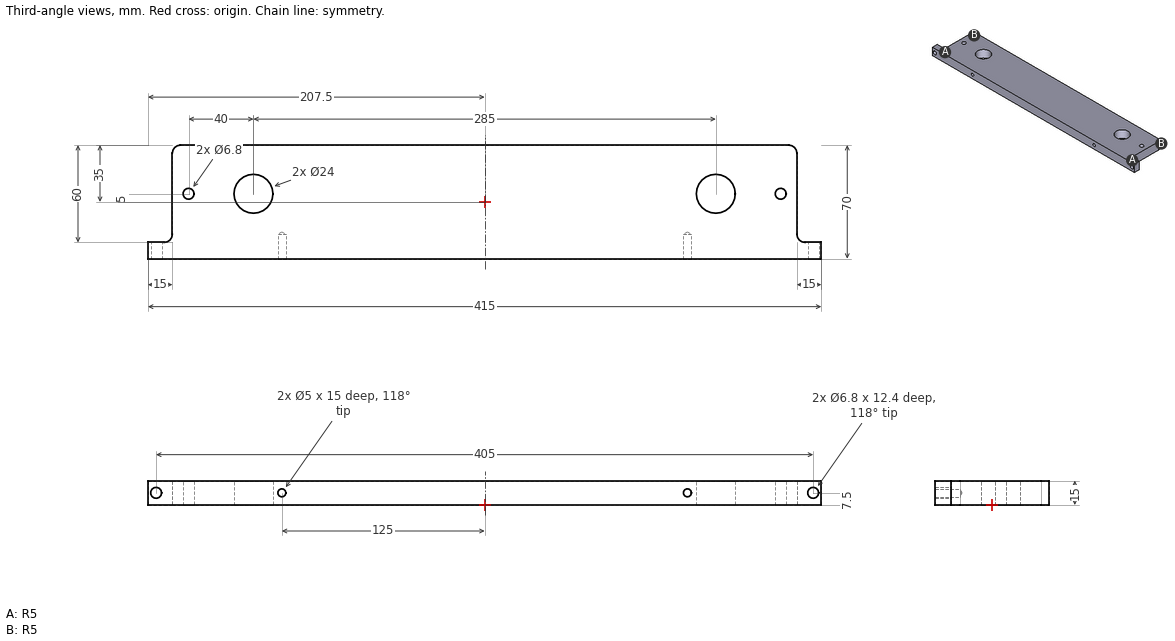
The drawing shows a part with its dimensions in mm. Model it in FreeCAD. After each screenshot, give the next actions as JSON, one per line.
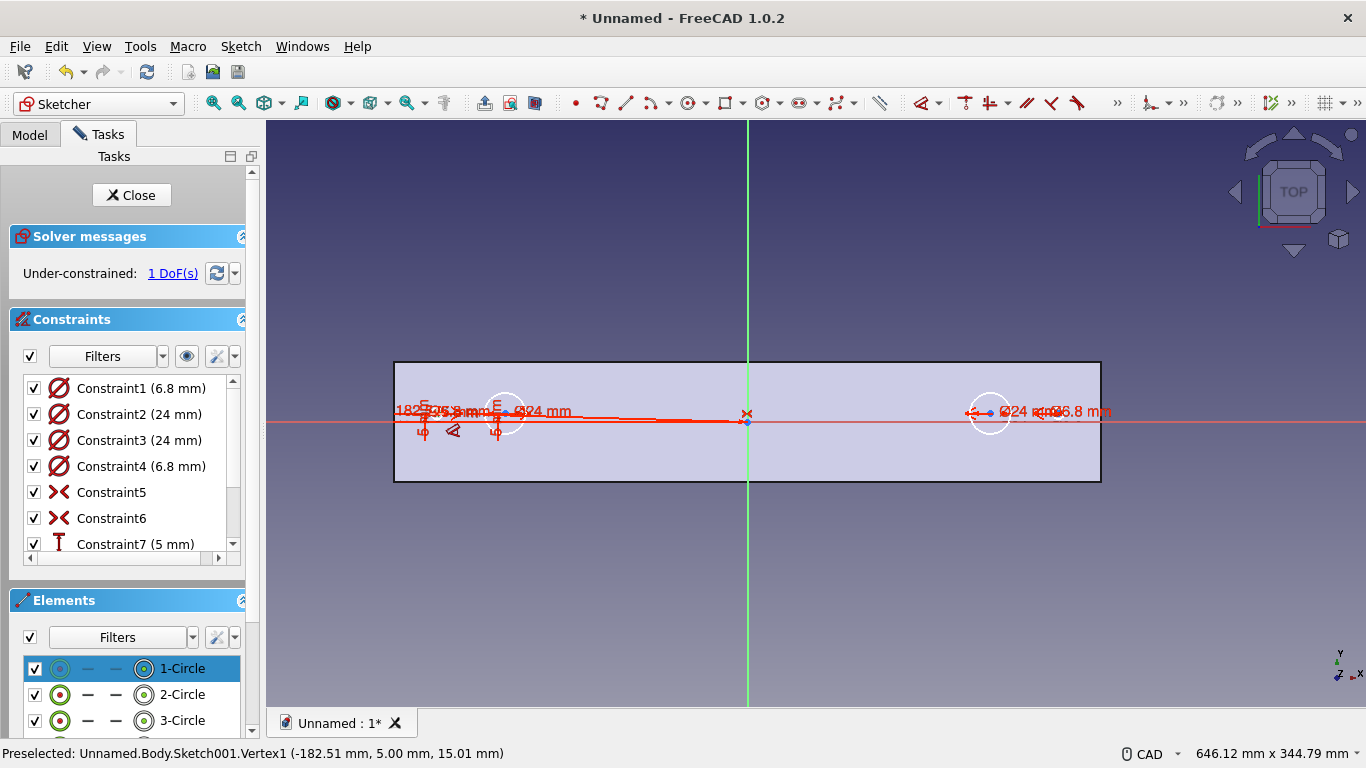
{"action": "left_click", "coordinate": [505, 414]}
{"action": "left_click", "coordinate": [471, 448]}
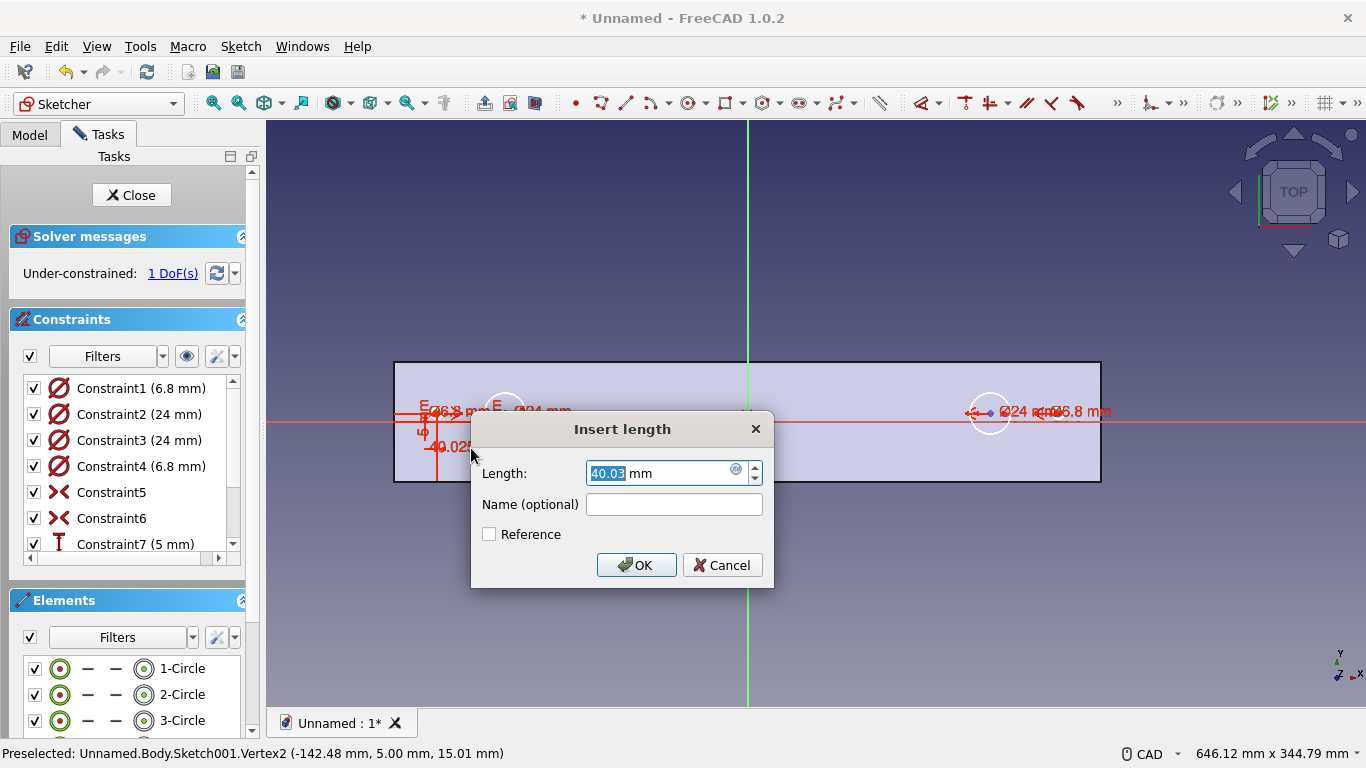
{"action": "type", "text": "40"}
{"action": "key", "text": "Return"}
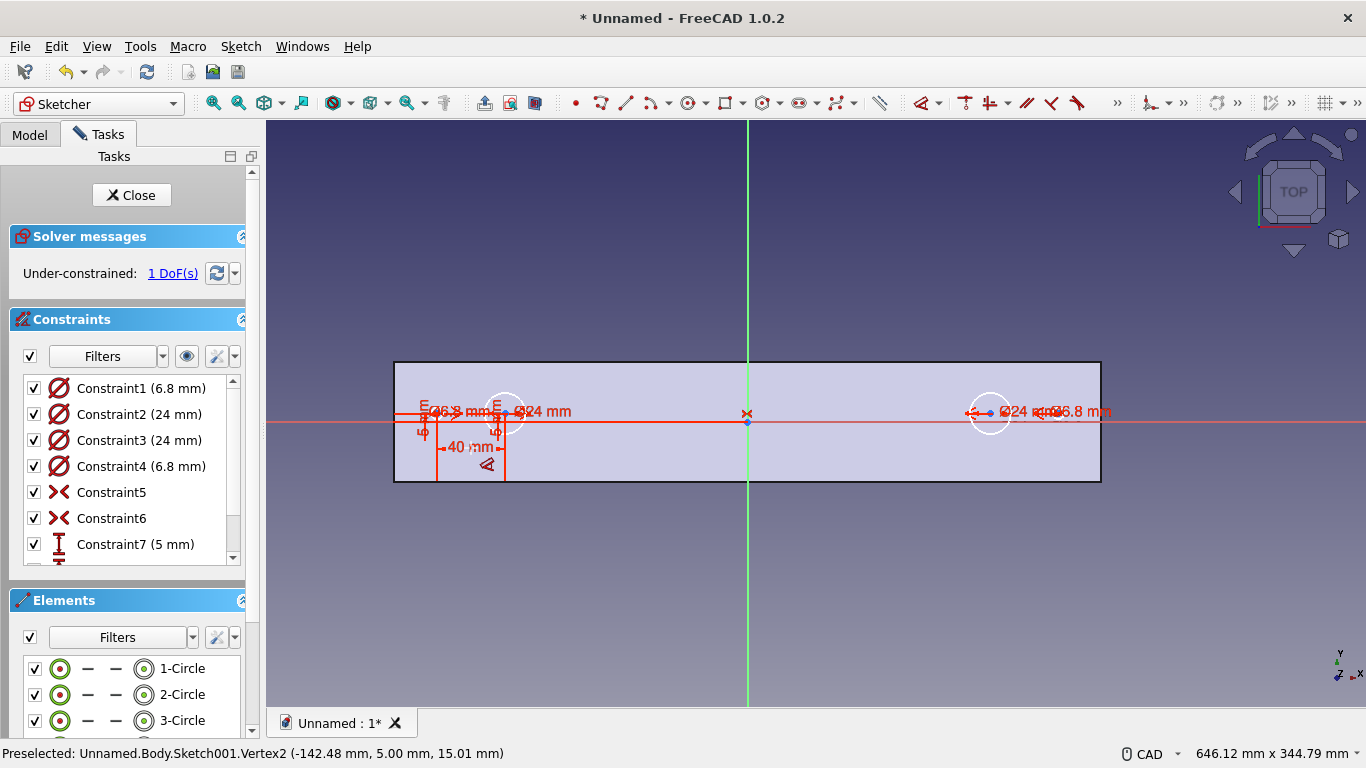
{"action": "left_click", "coordinate": [505, 414]}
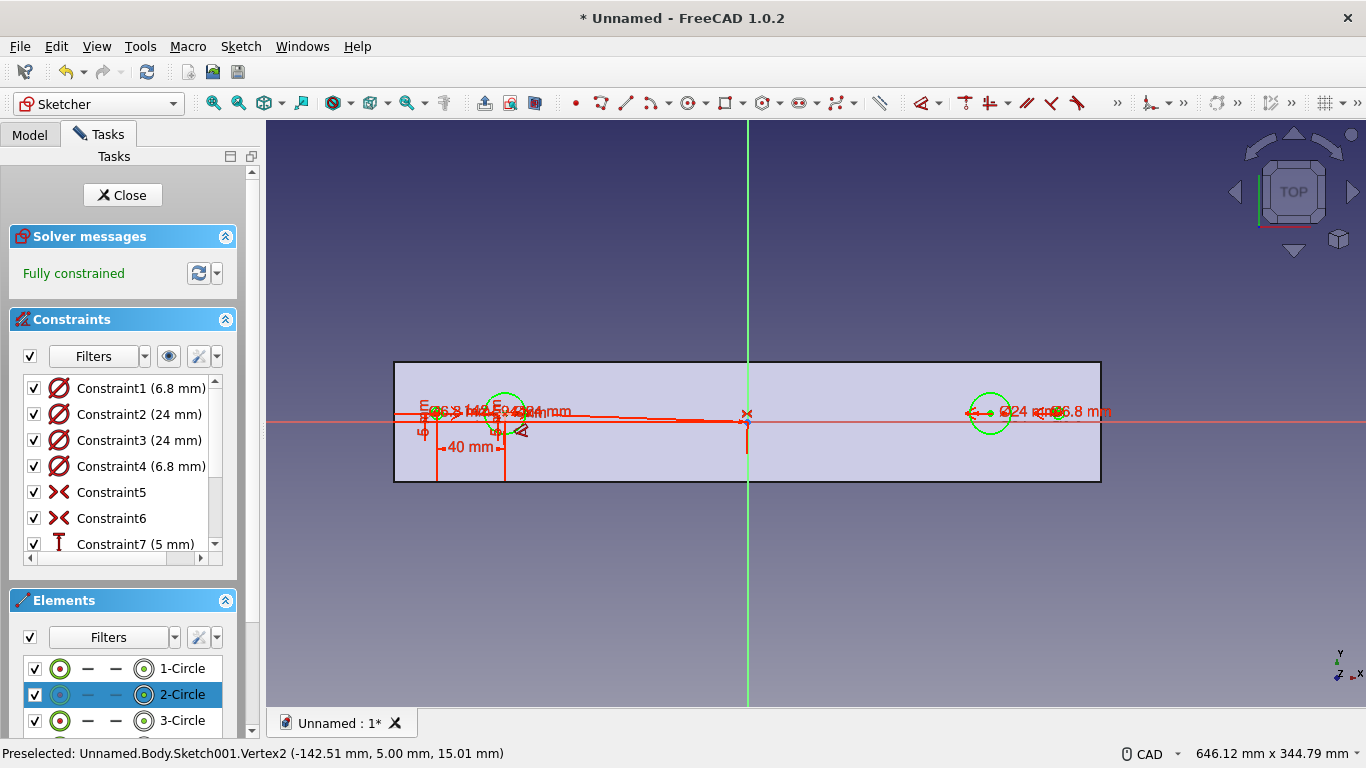
{"action": "left_click", "coordinate": [990, 414]}
{"action": "left_click", "coordinate": [636, 448]}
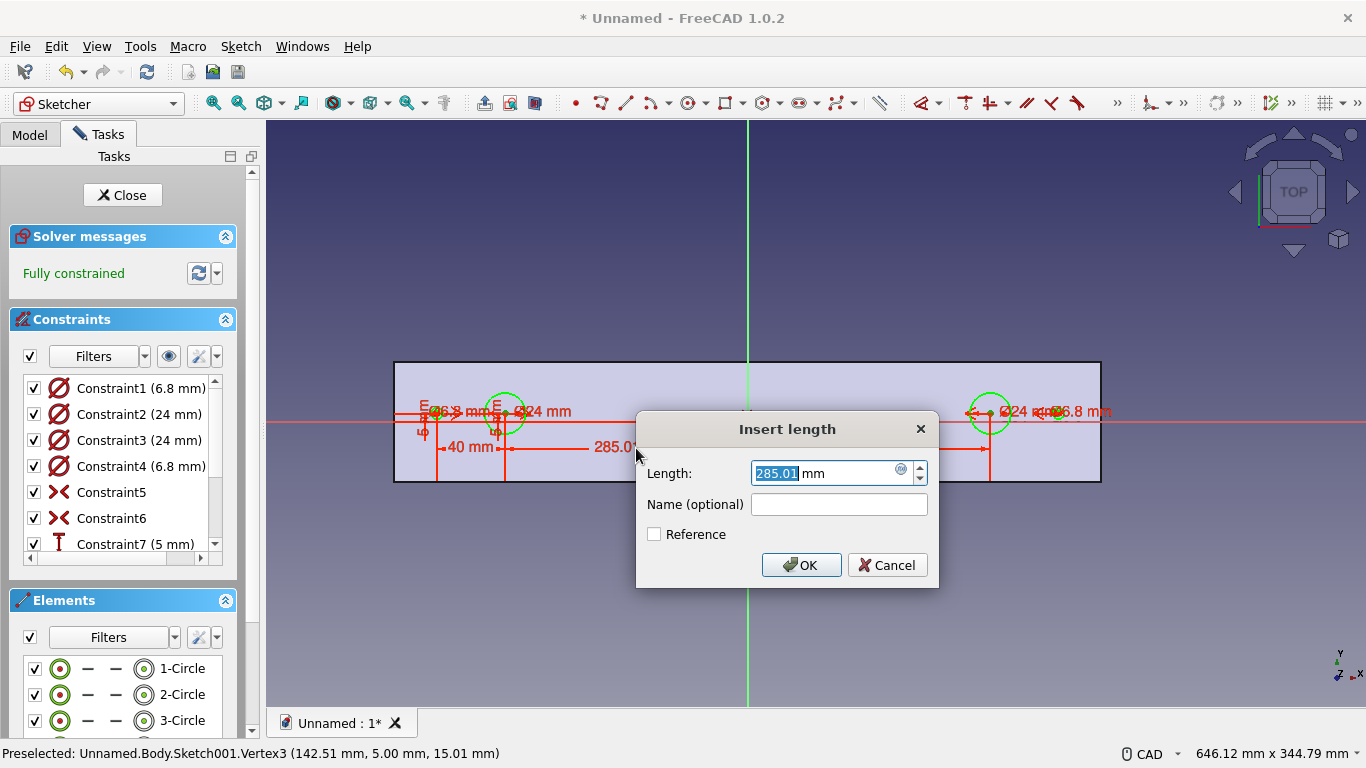
{"action": "type", "text": "285"}
{"action": "key", "text": "Return"}
{"action": "key", "text": "Escape"}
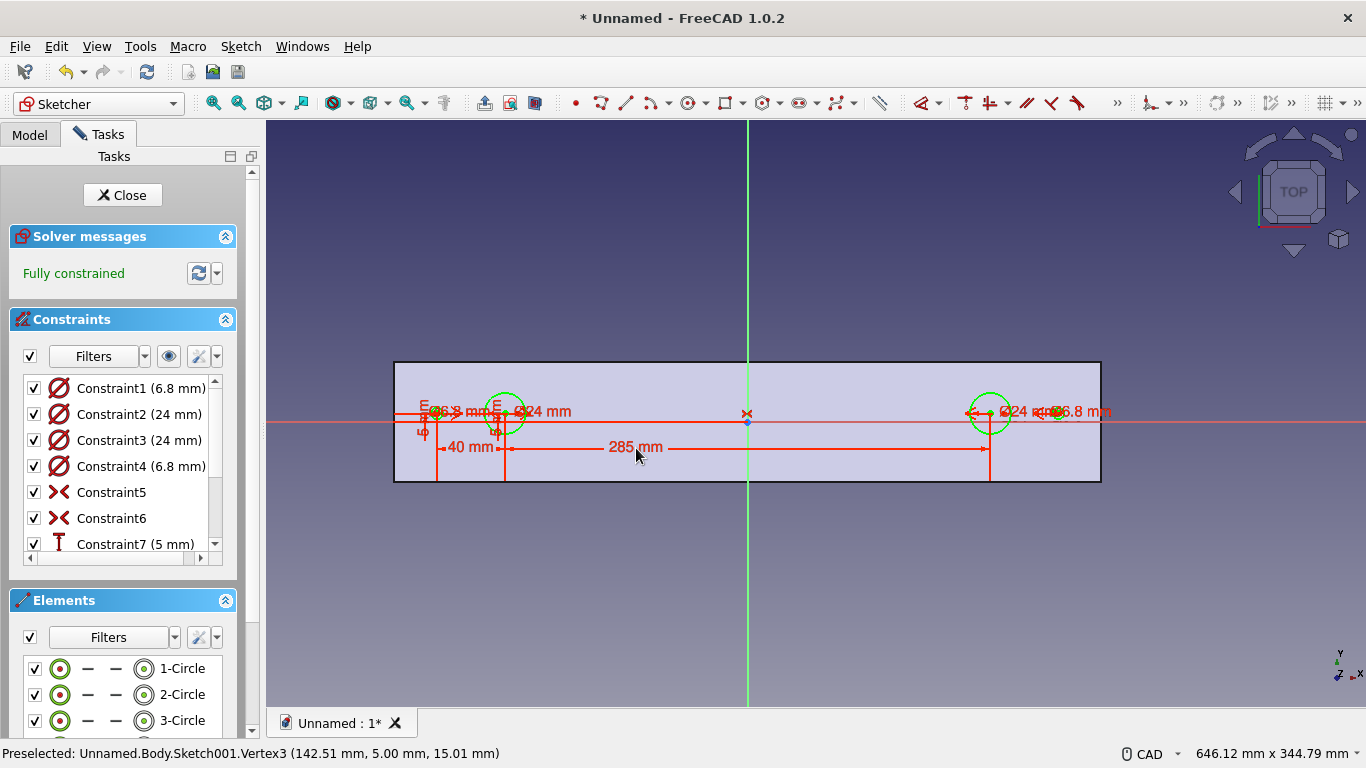
{"action": "left_click", "coordinate": [123, 195]}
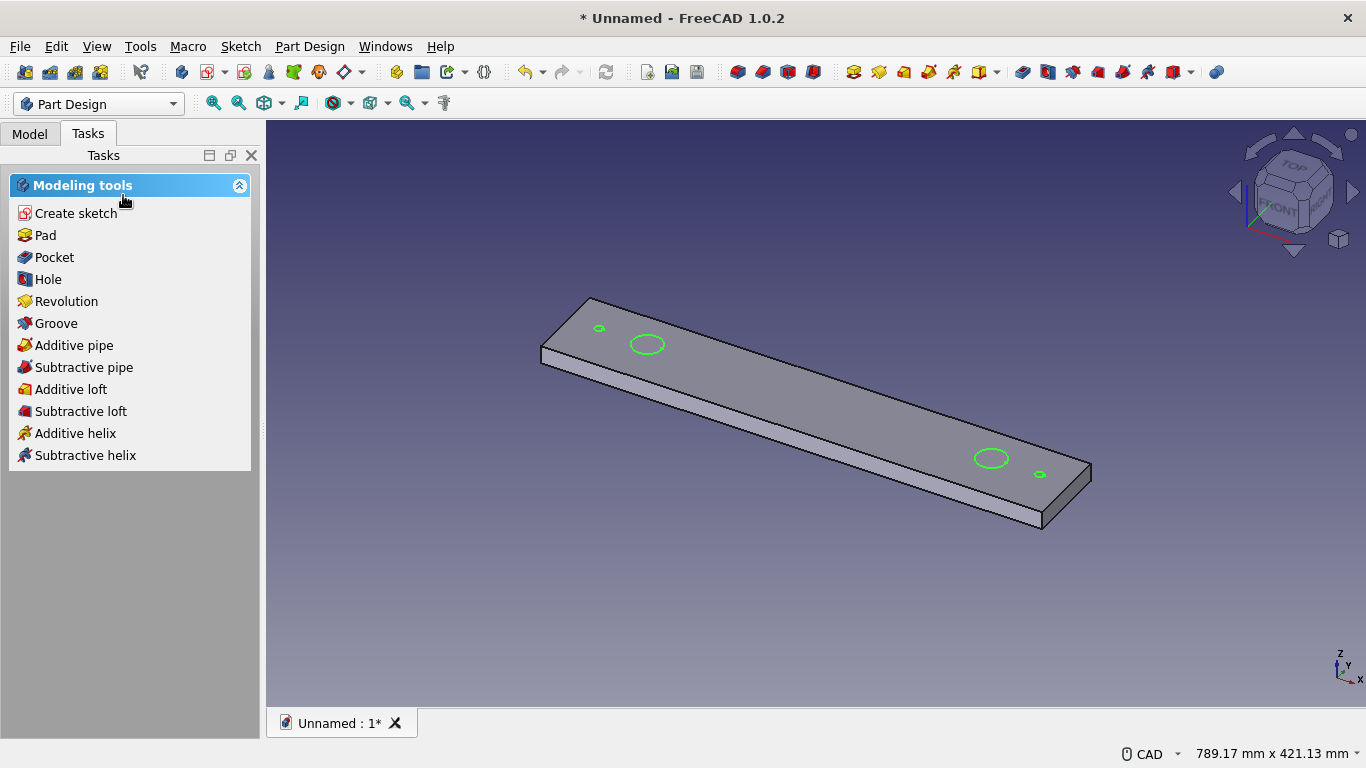
{"action": "left_click", "coordinate": [1023, 72]}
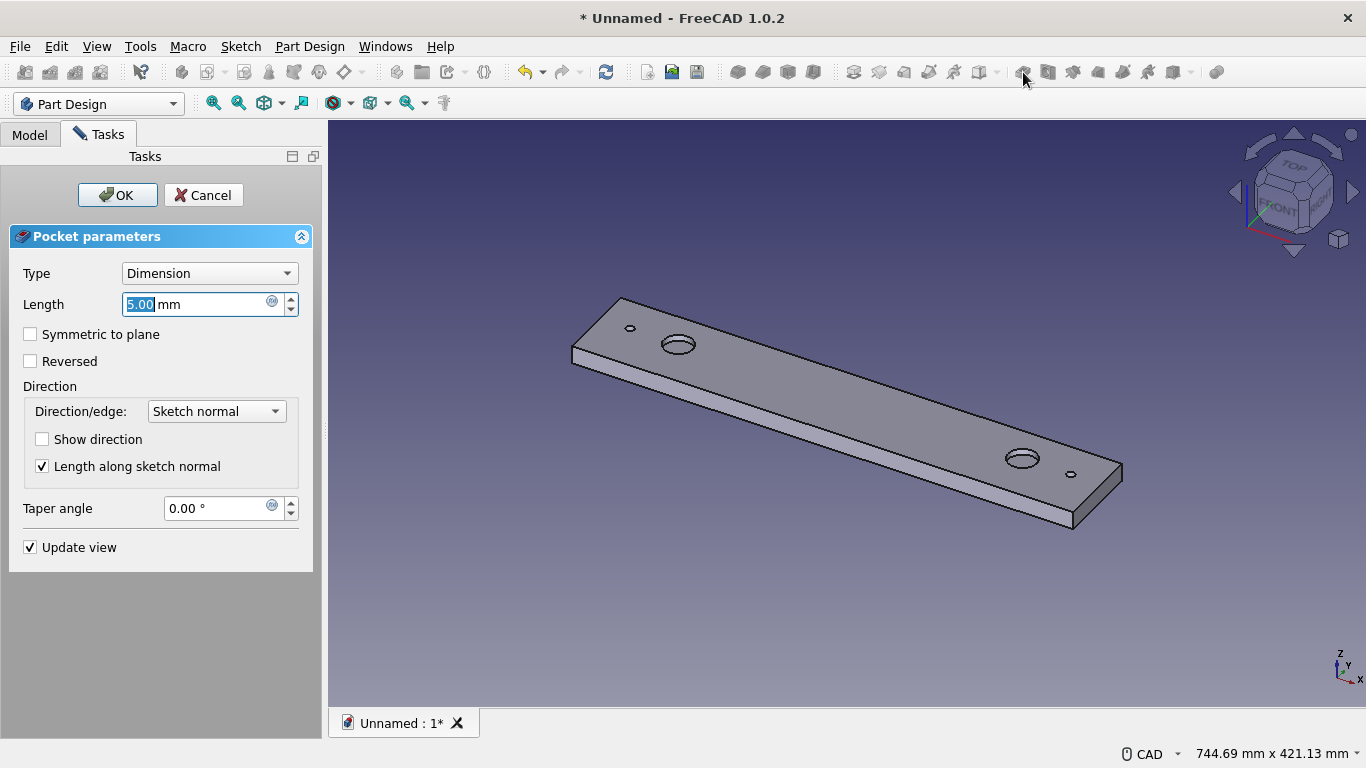
{"action": "left_click", "coordinate": [210, 274]}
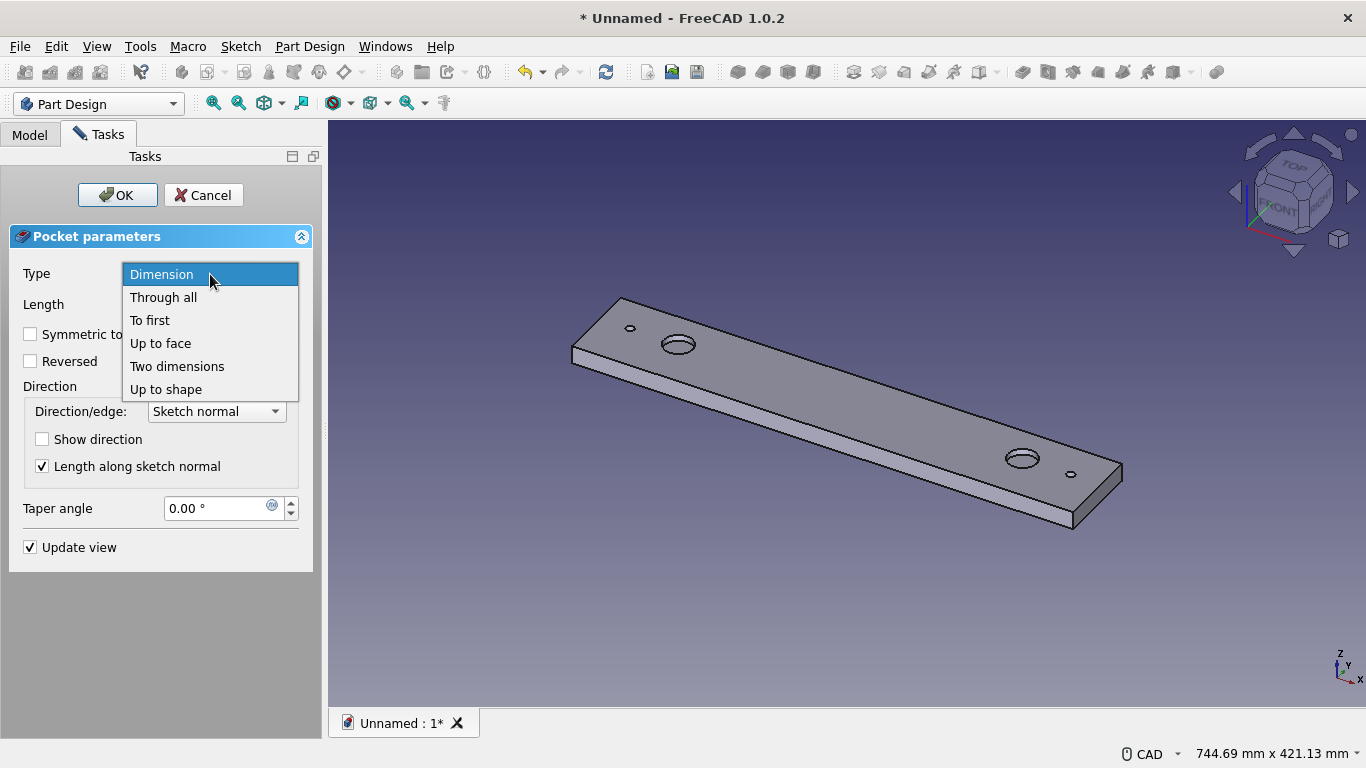
{"action": "left_click", "coordinate": [208, 298]}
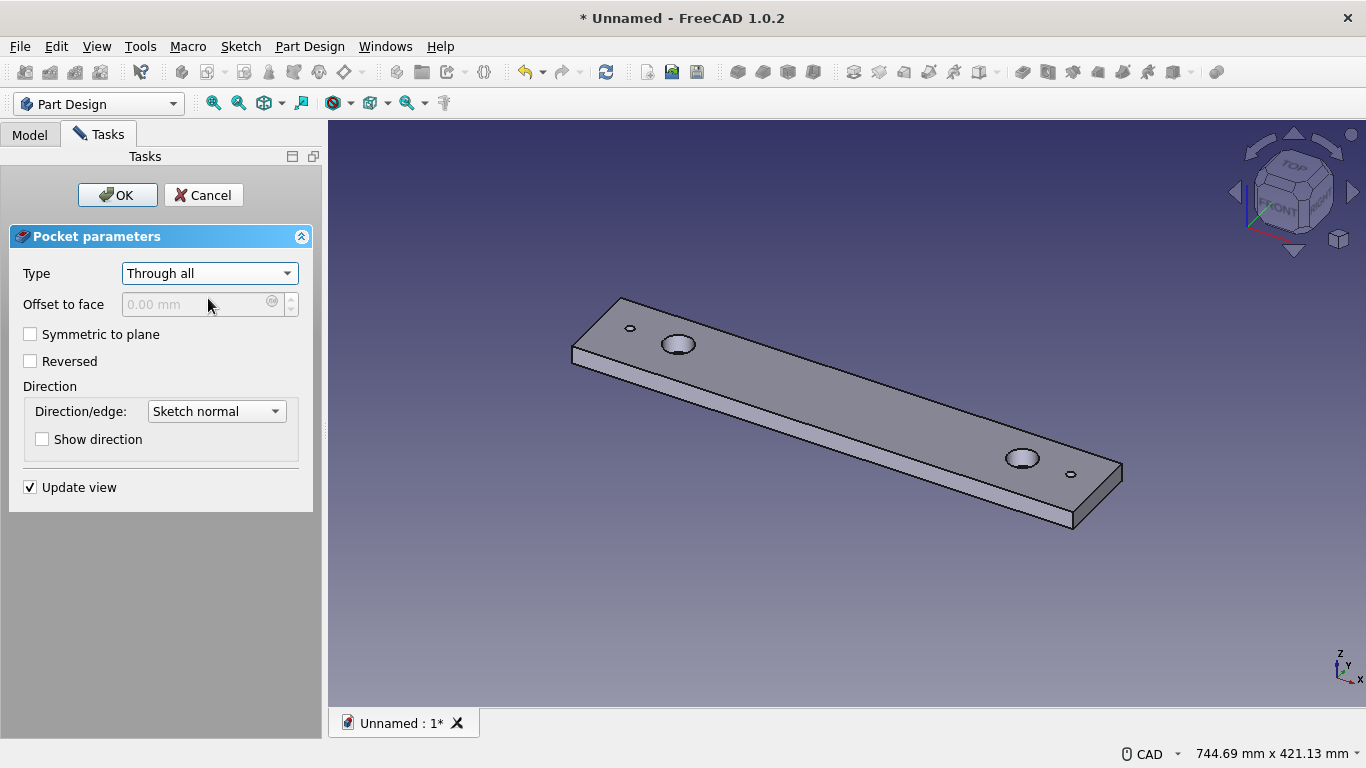
{"action": "left_click", "coordinate": [118, 195]}